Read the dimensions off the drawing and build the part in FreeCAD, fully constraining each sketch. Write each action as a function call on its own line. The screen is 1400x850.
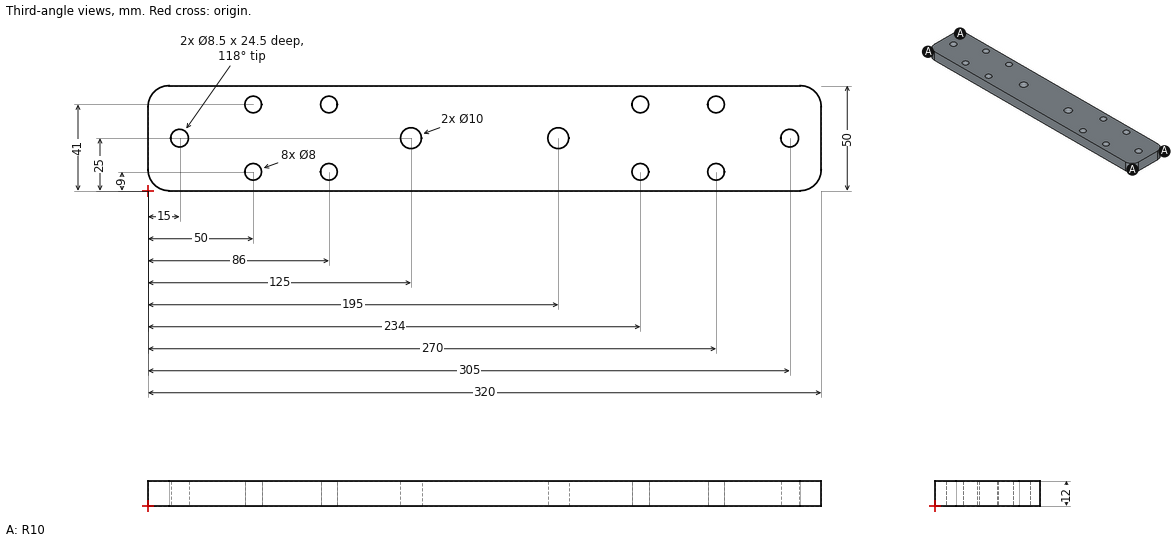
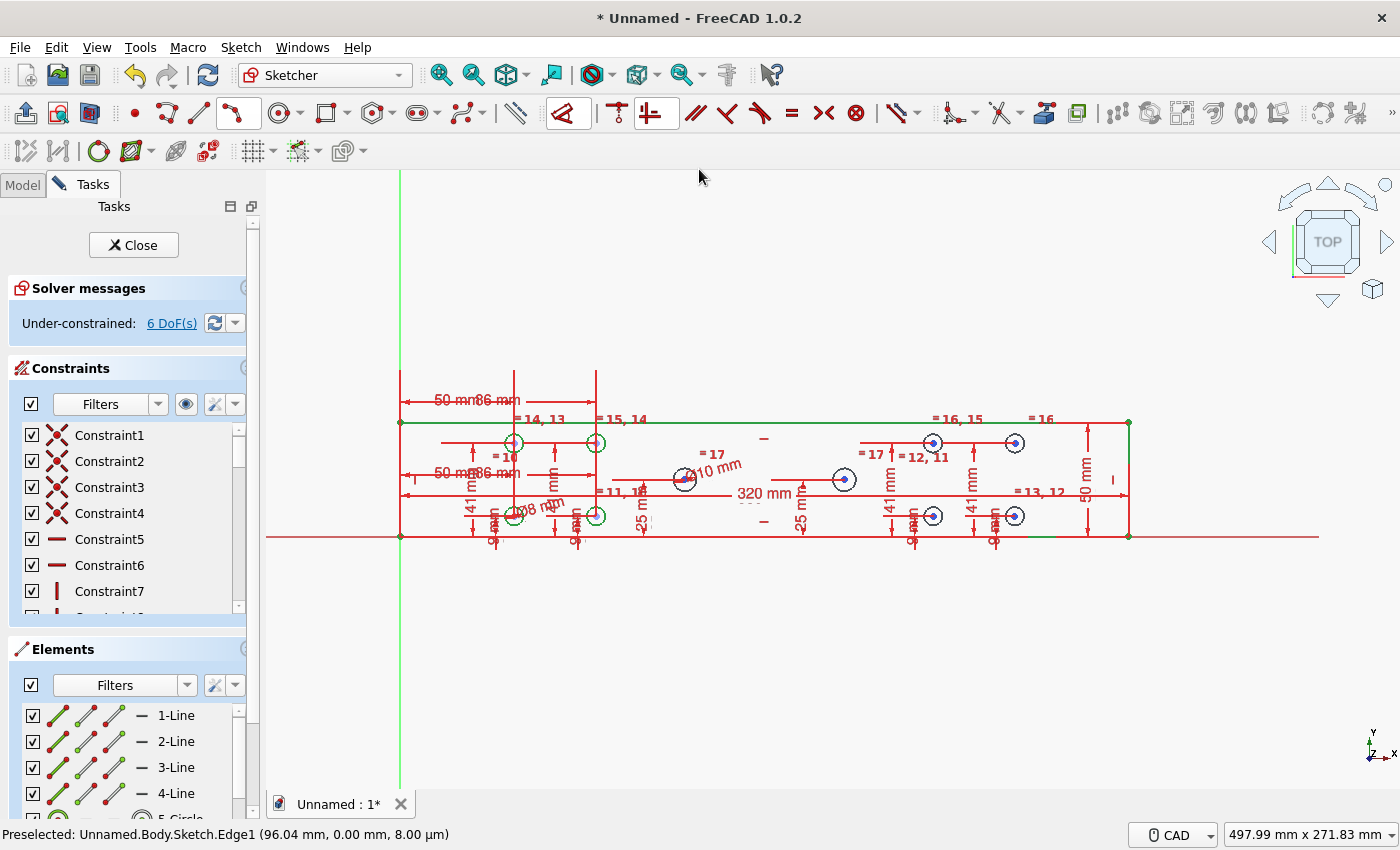
click(933, 516)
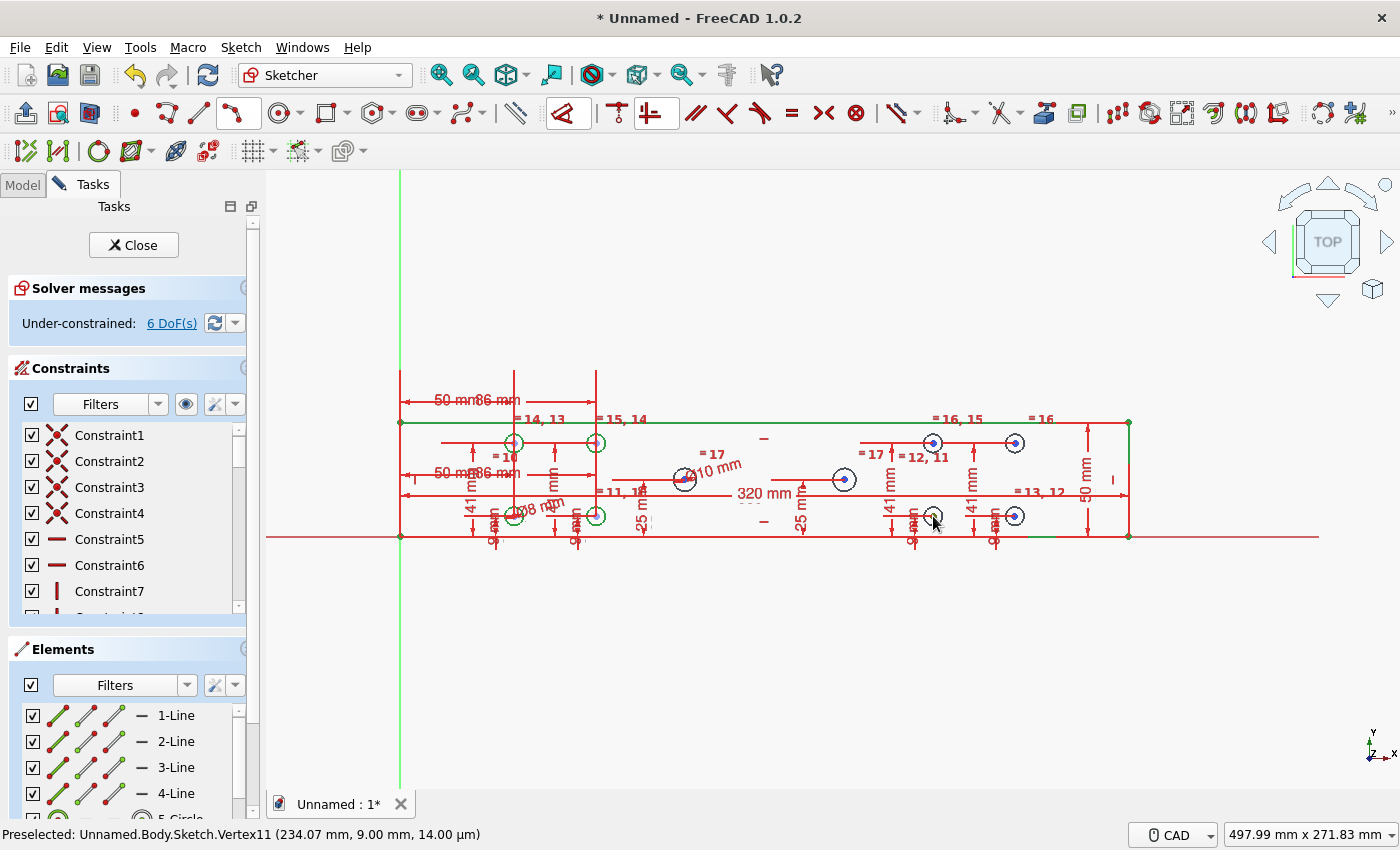
key(l)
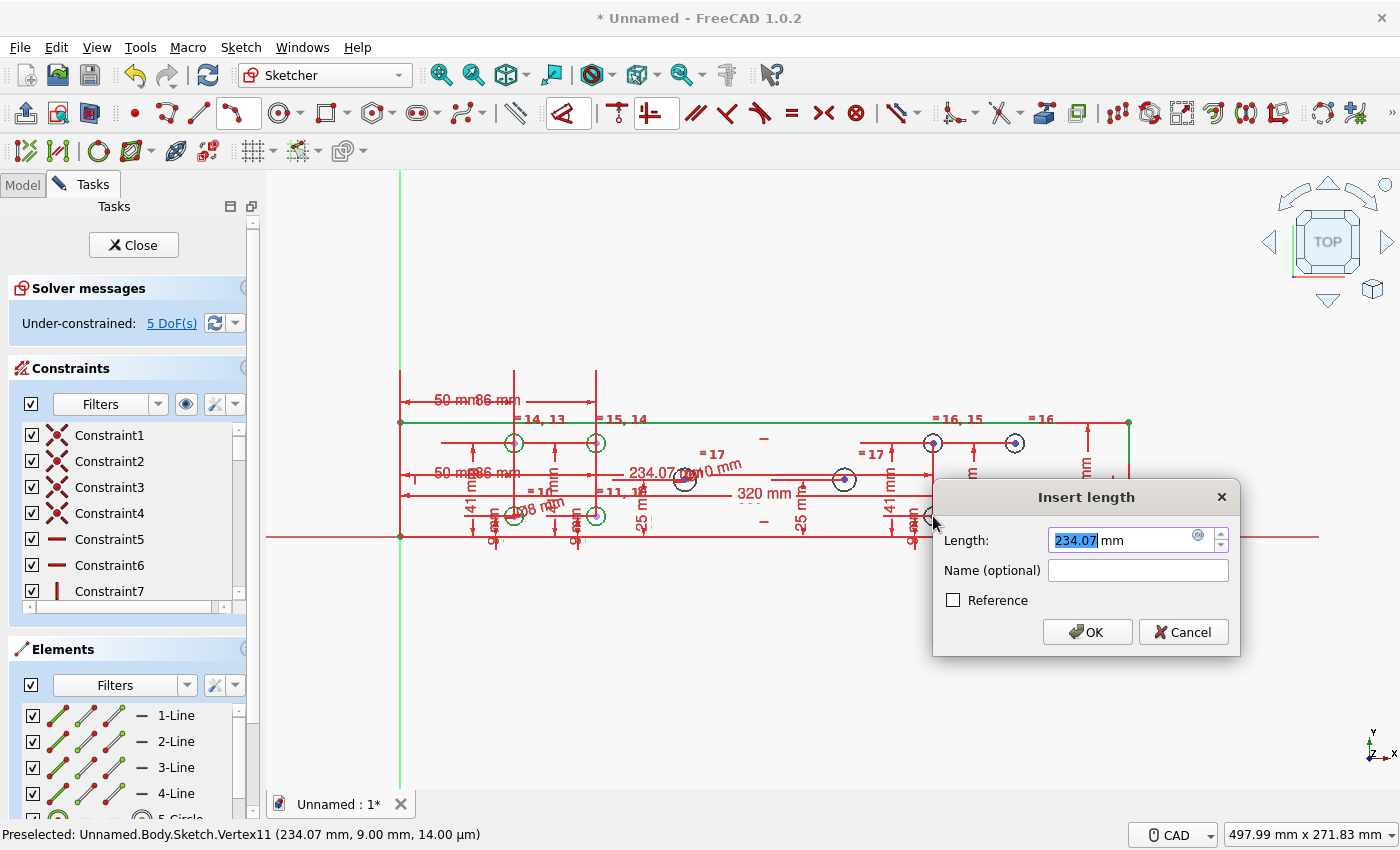
text(234)
key(Return)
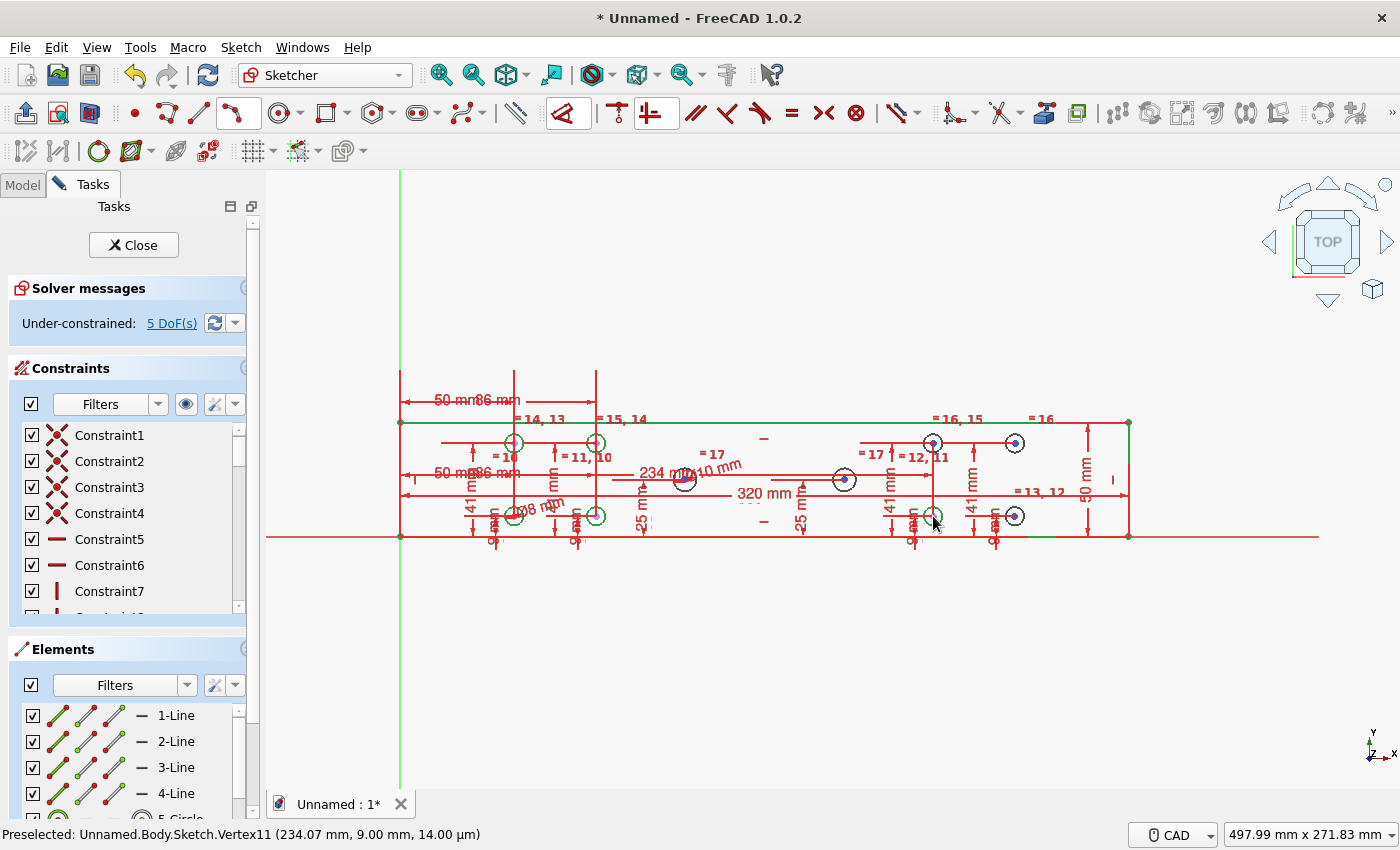
click(1015, 516)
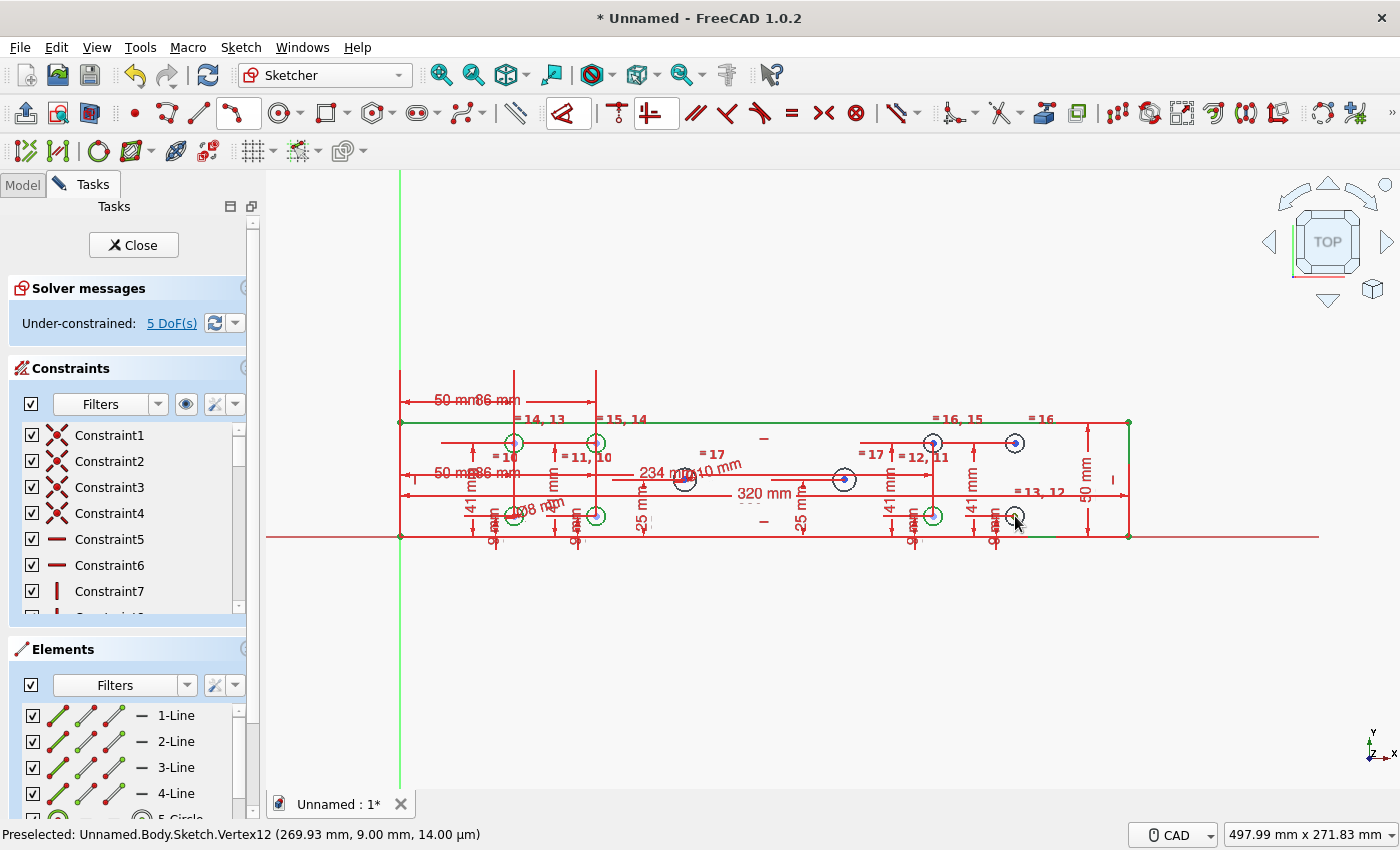
key(l)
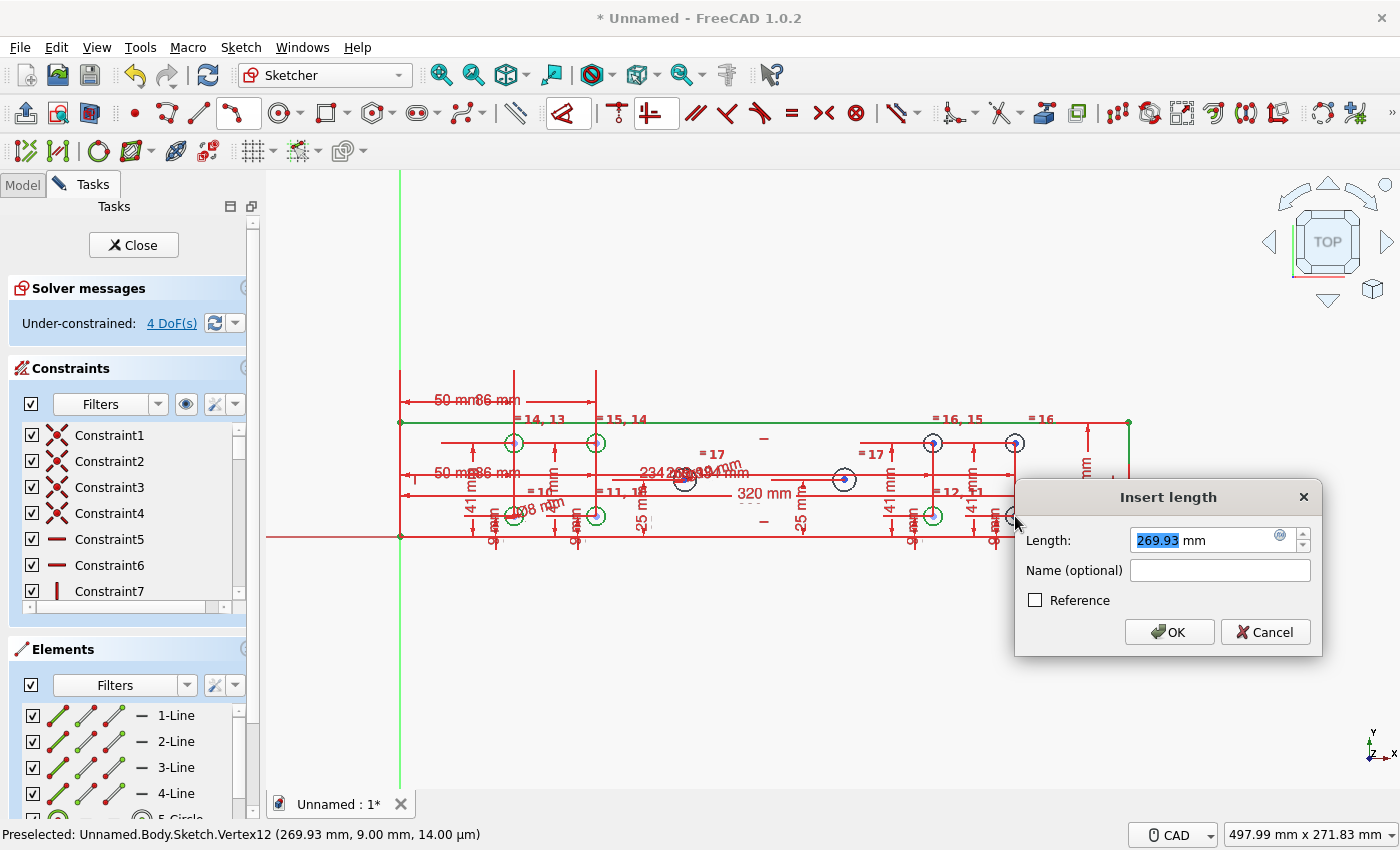
text(270)
key(Return)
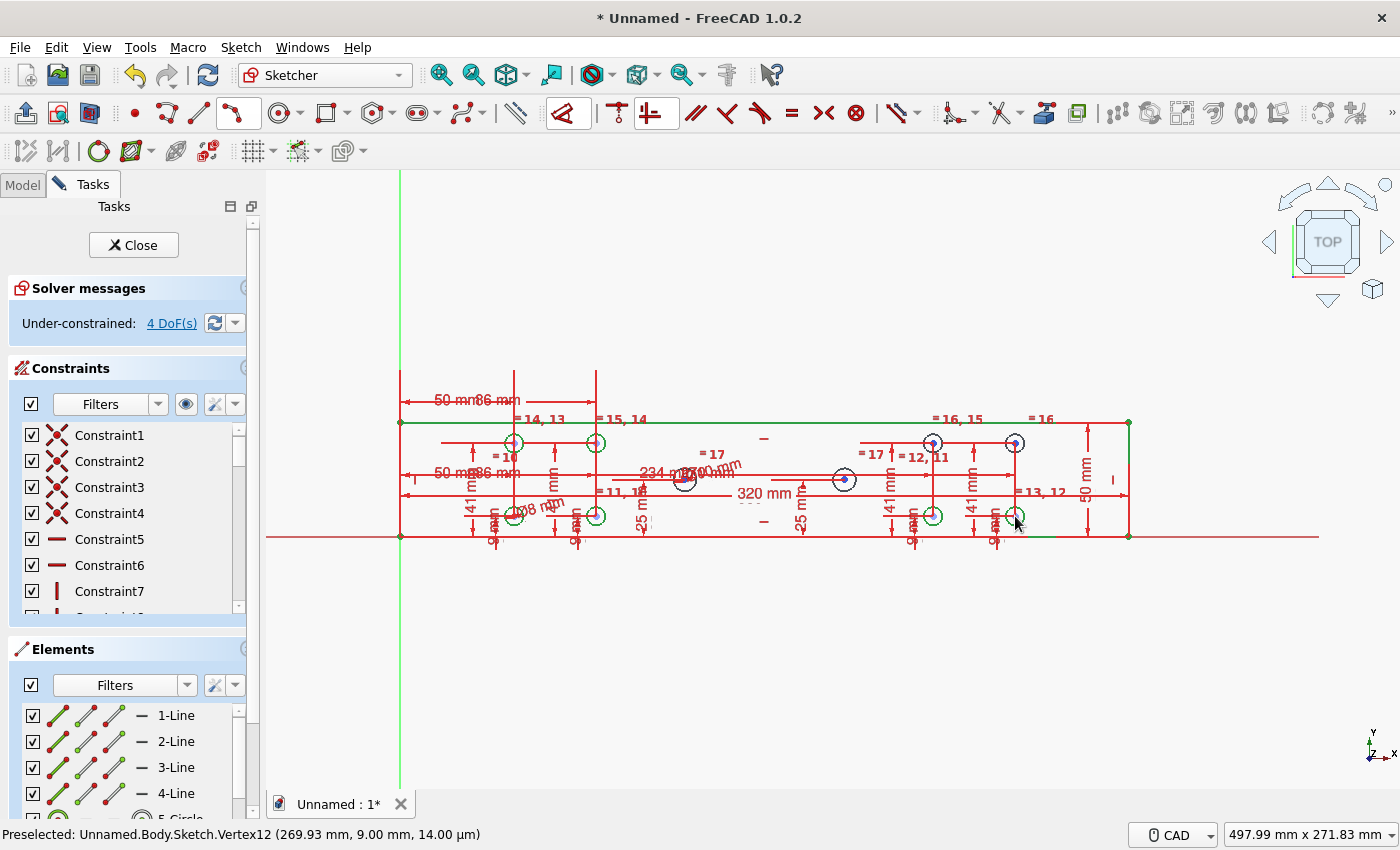
click(685, 480)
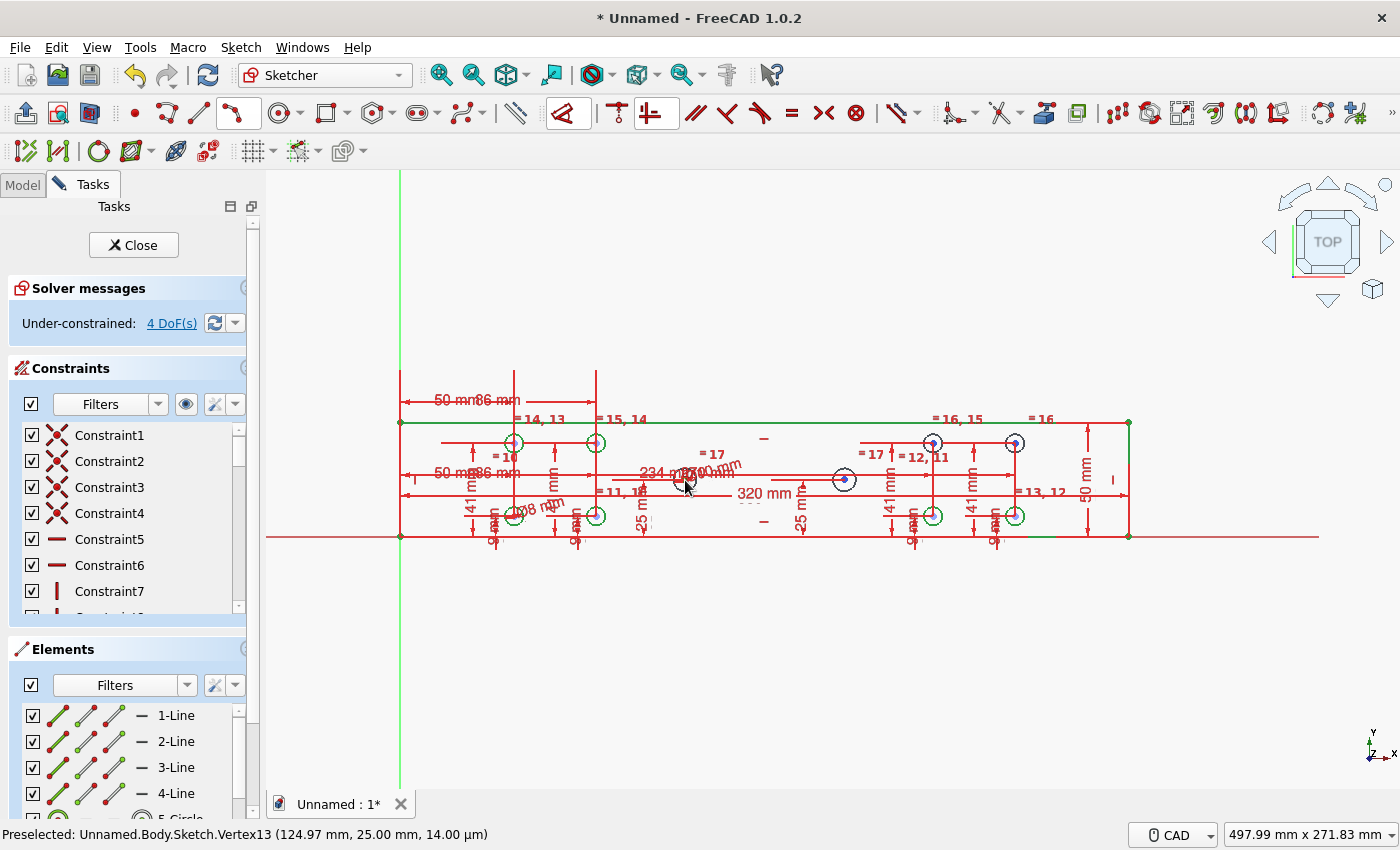
key(l)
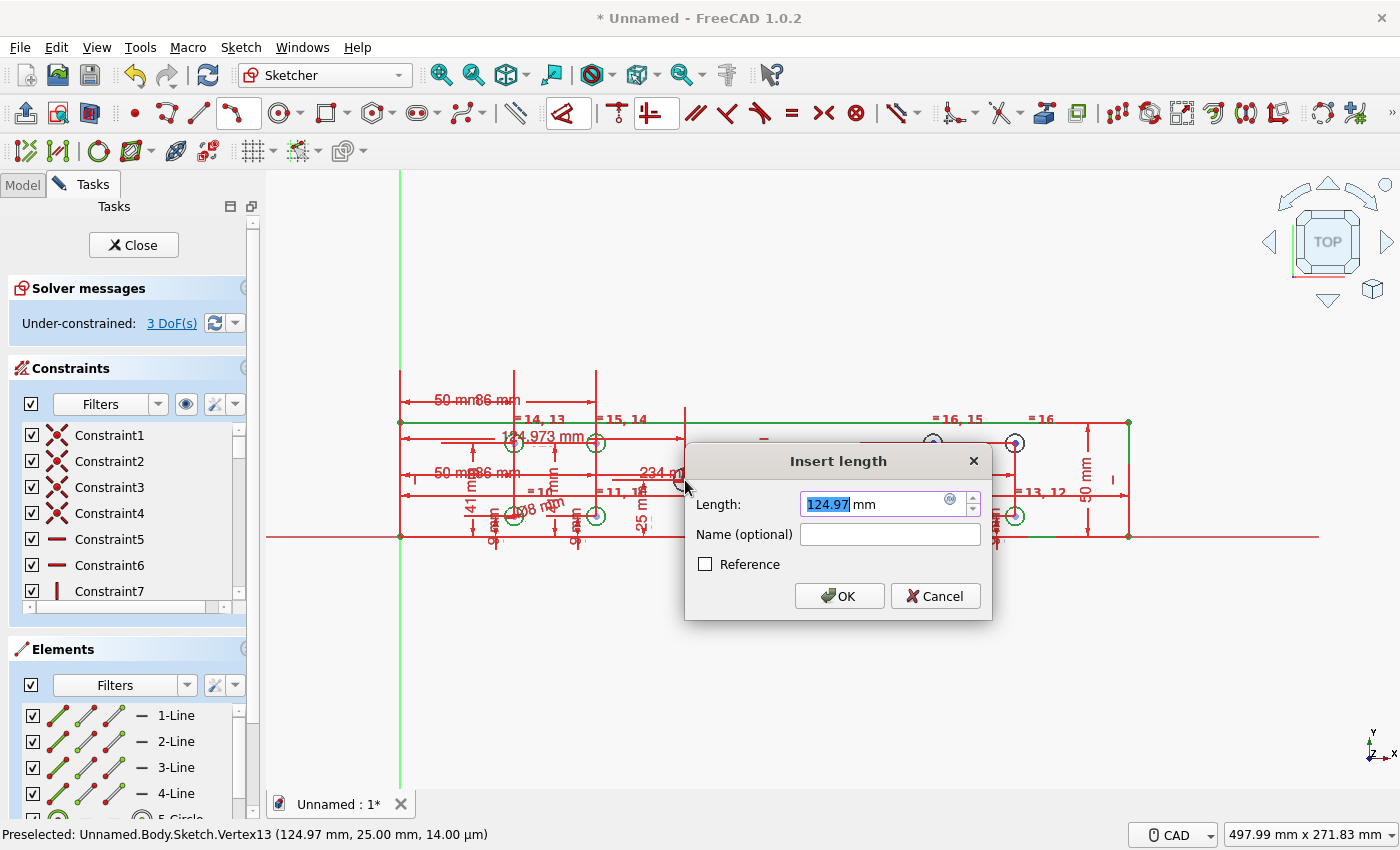
text(125)
key(Return)